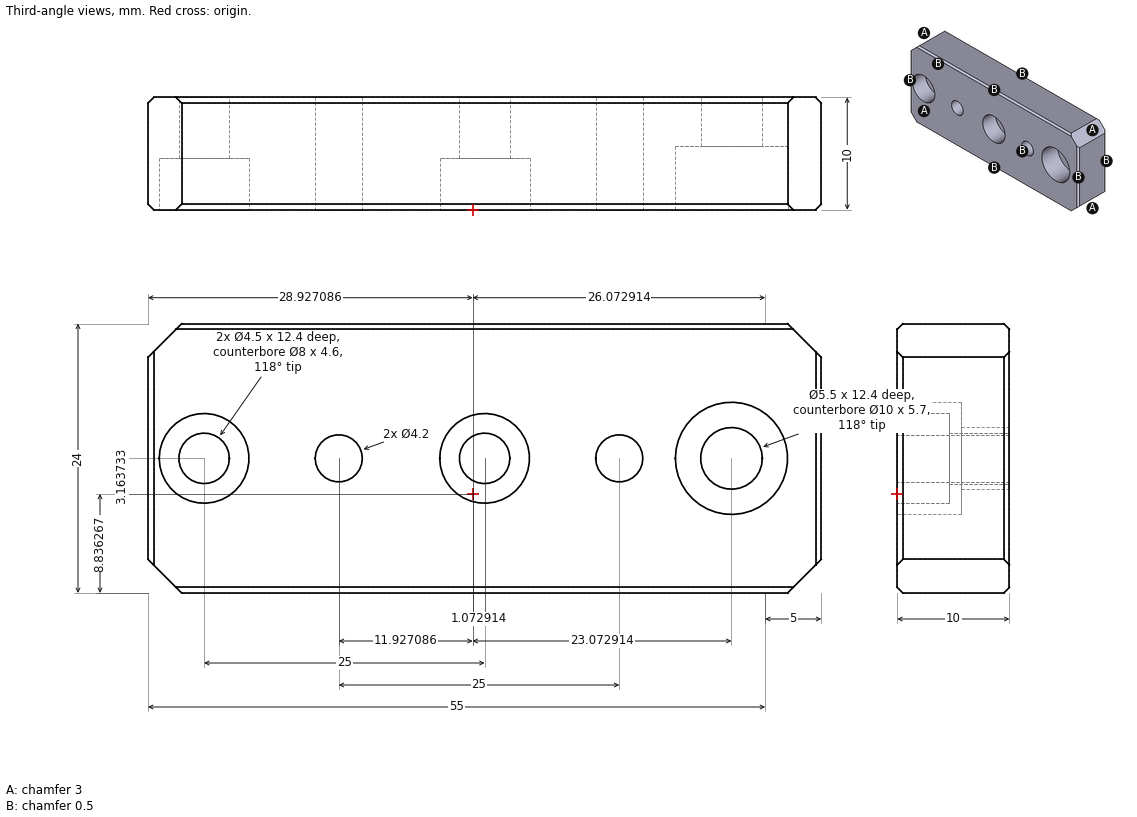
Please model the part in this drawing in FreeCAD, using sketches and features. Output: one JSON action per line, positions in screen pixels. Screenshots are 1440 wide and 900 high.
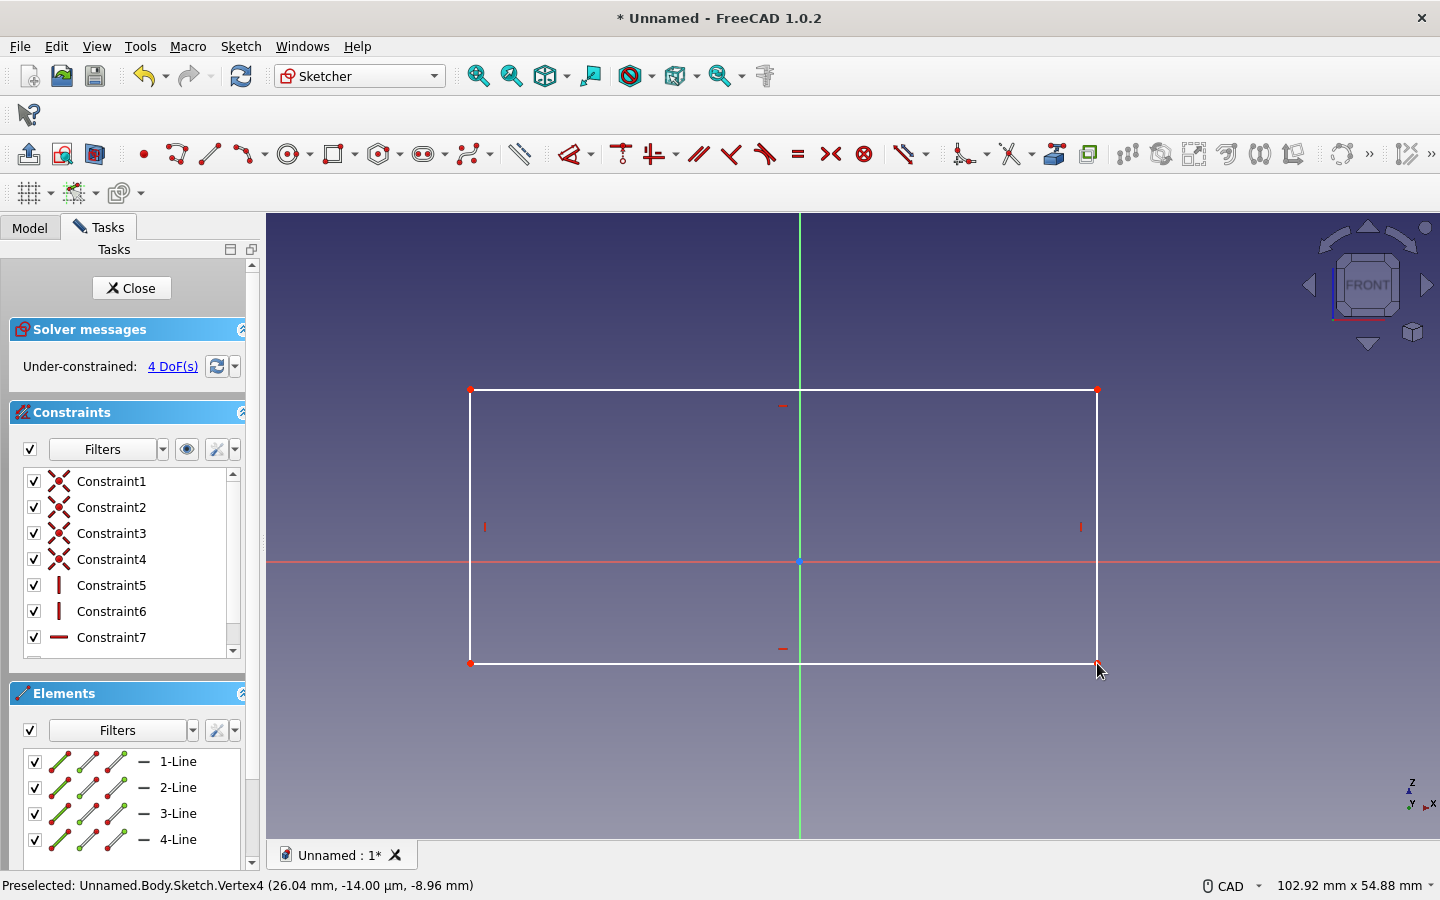
{"action": "key", "text": "d"}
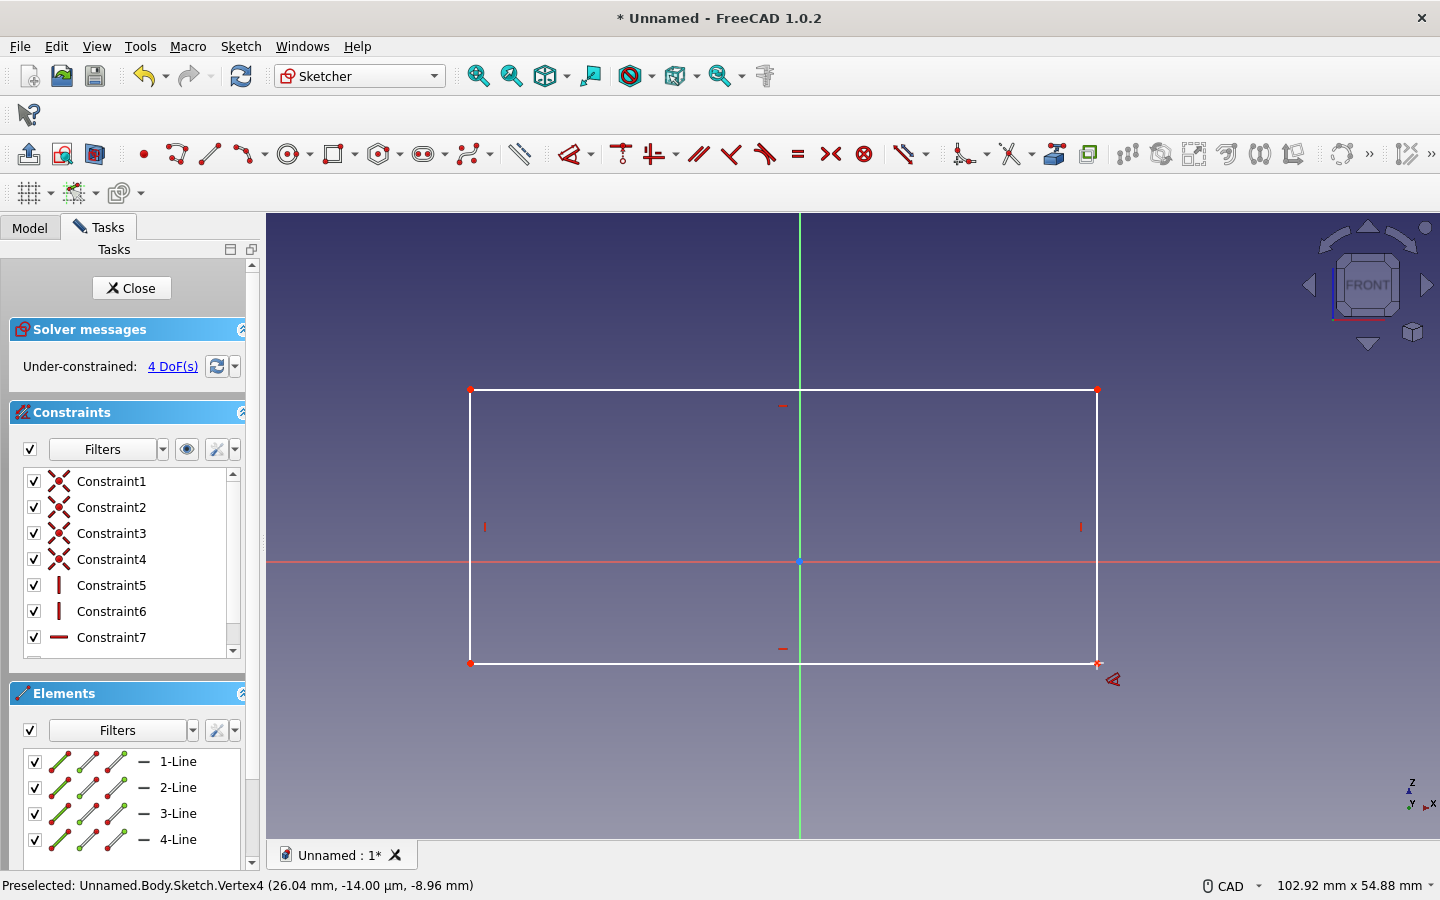
{"action": "left_click", "coordinate": [470, 472]}
{"action": "left_click", "coordinate": [436, 527]}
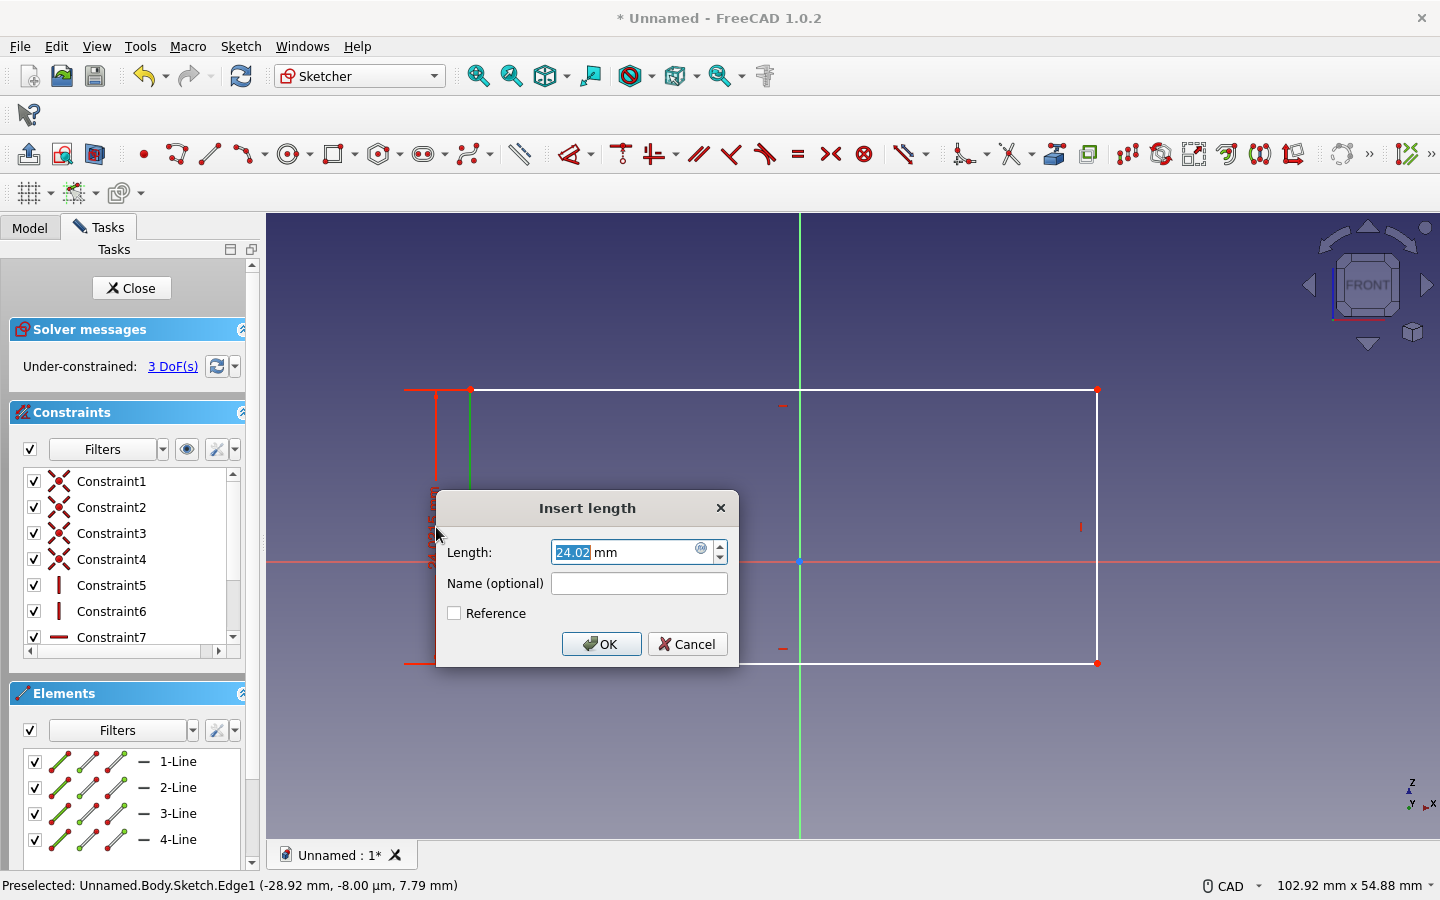
{"action": "type", "text": "24"}
{"action": "key", "text": "Return"}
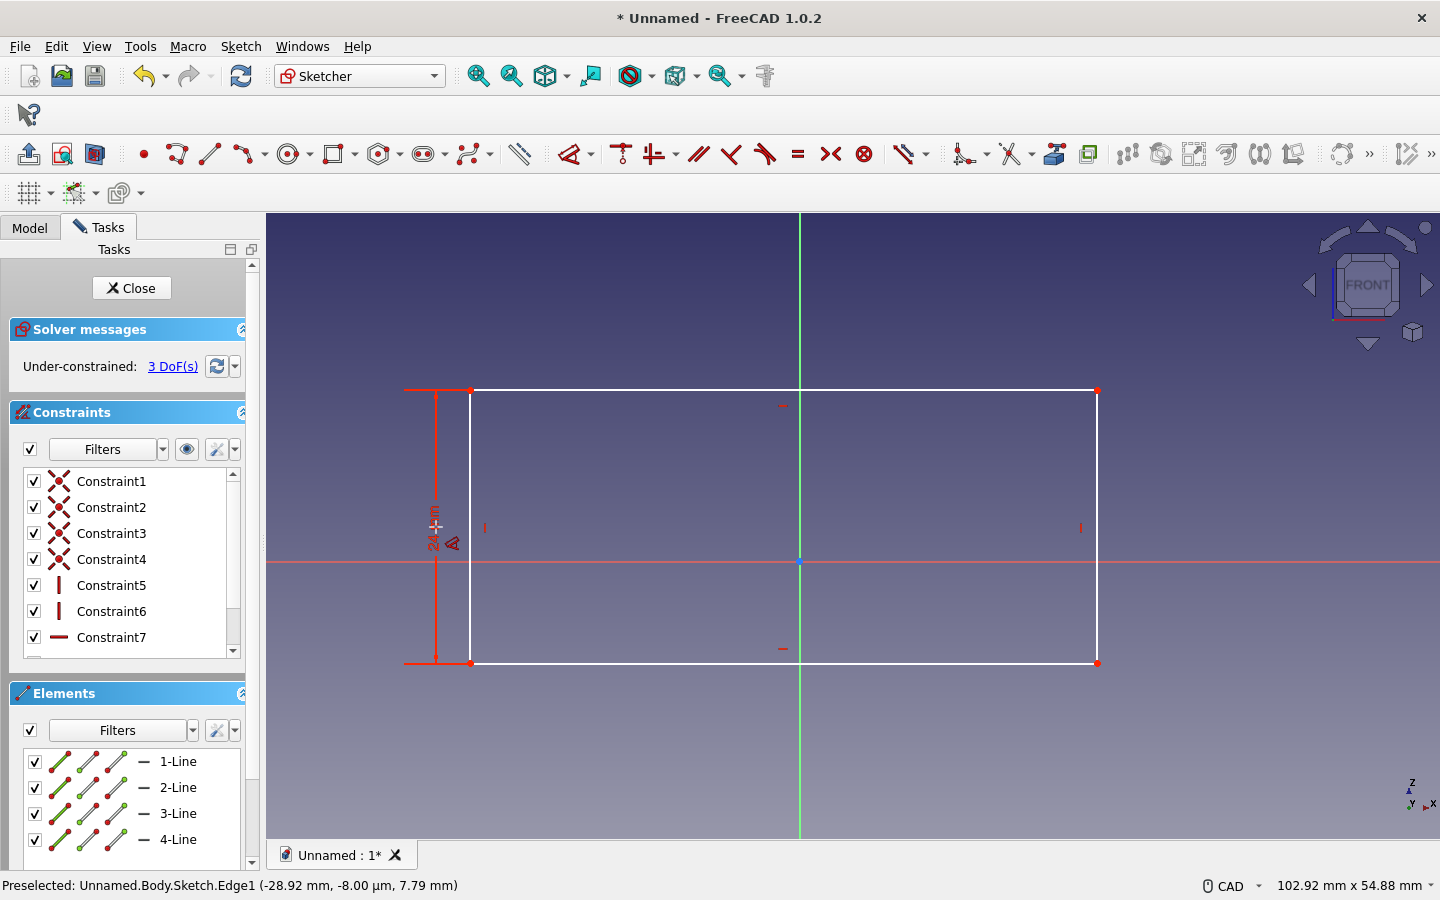
{"action": "left_click", "coordinate": [658, 664]}
{"action": "left_click", "coordinate": [783, 698]}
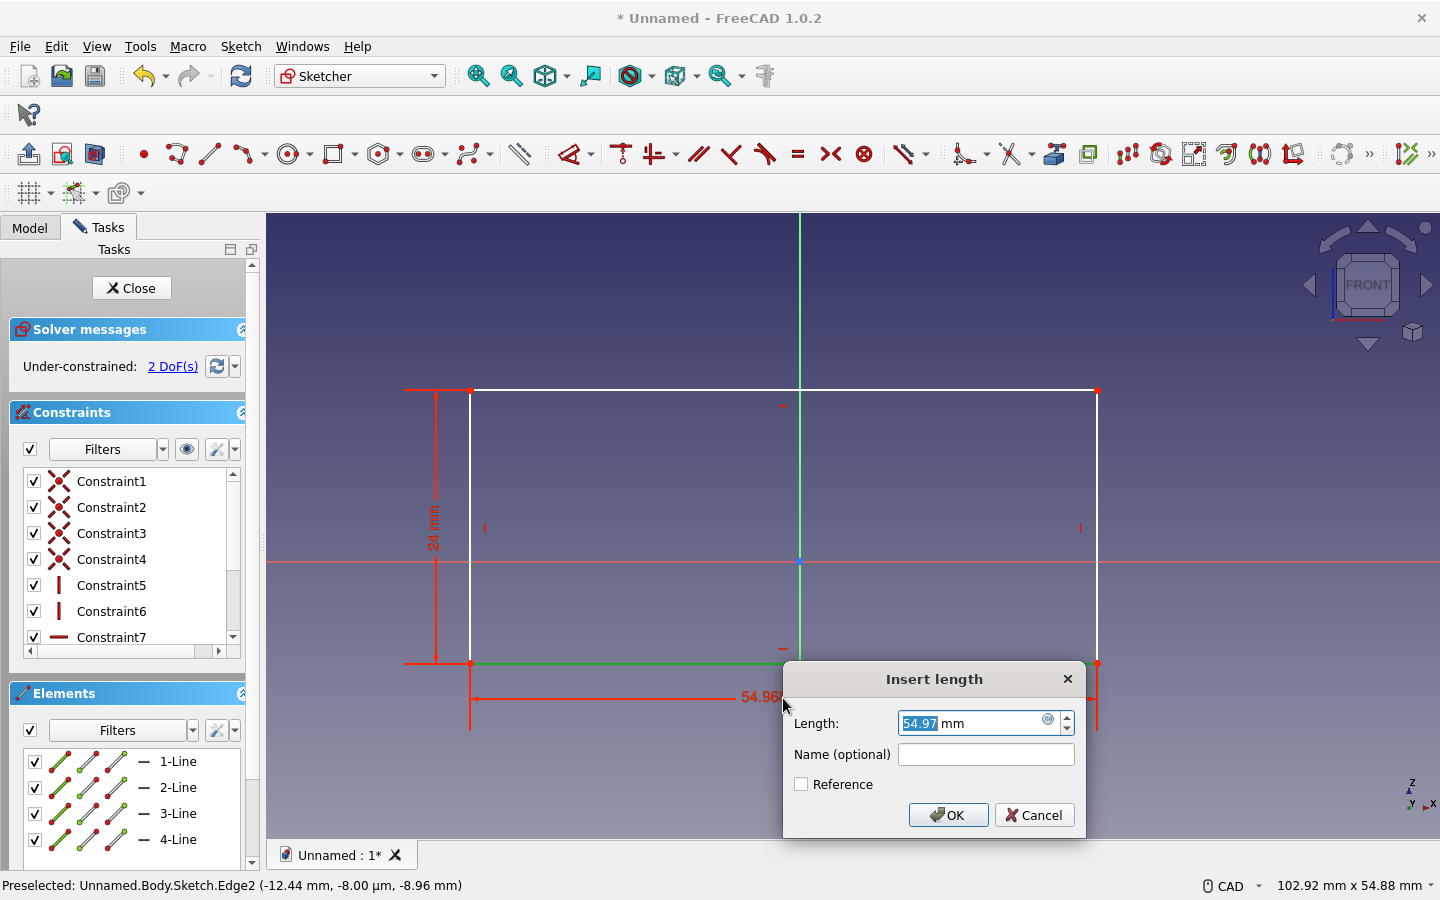
{"action": "type", "text": "55"}
{"action": "key", "text": "Return"}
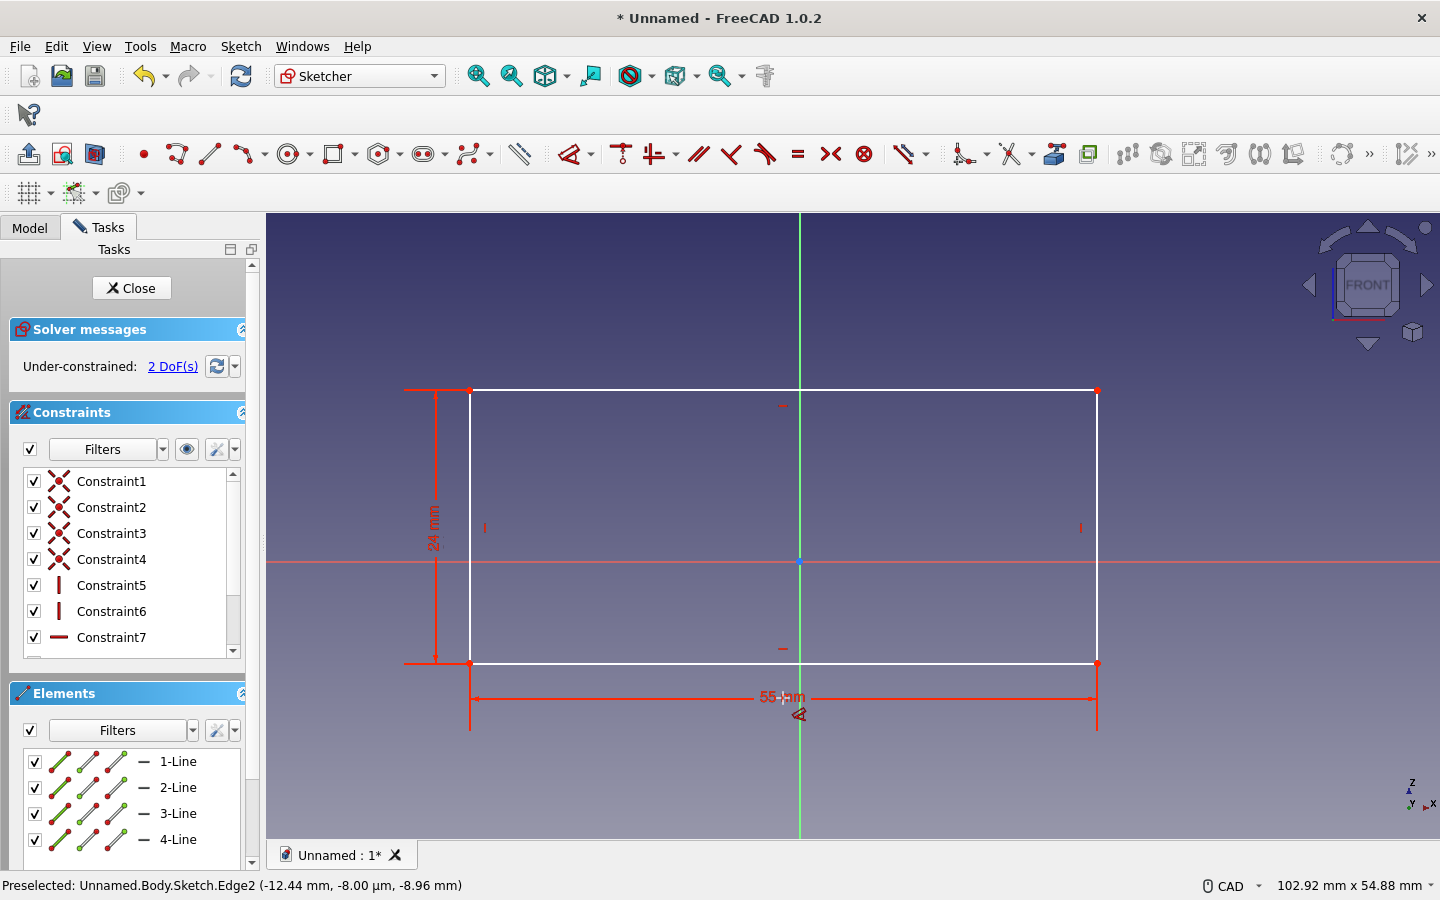
{"action": "left_click", "coordinate": [470, 664]}
{"action": "left_click", "coordinate": [436, 613]}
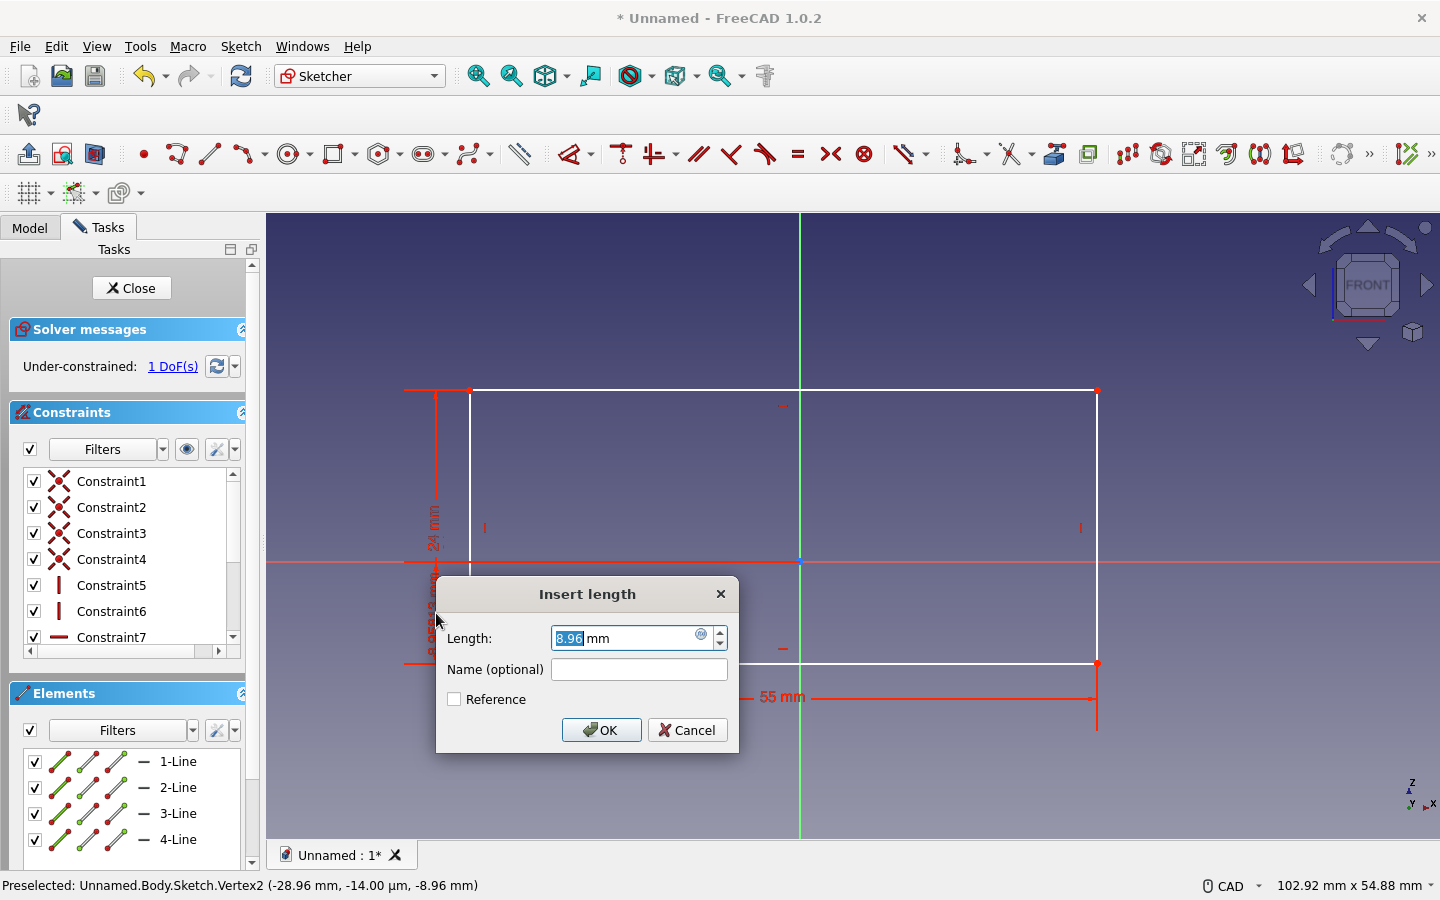
{"action": "type", "text": "8.836267"}
{"action": "key", "text": "Return"}